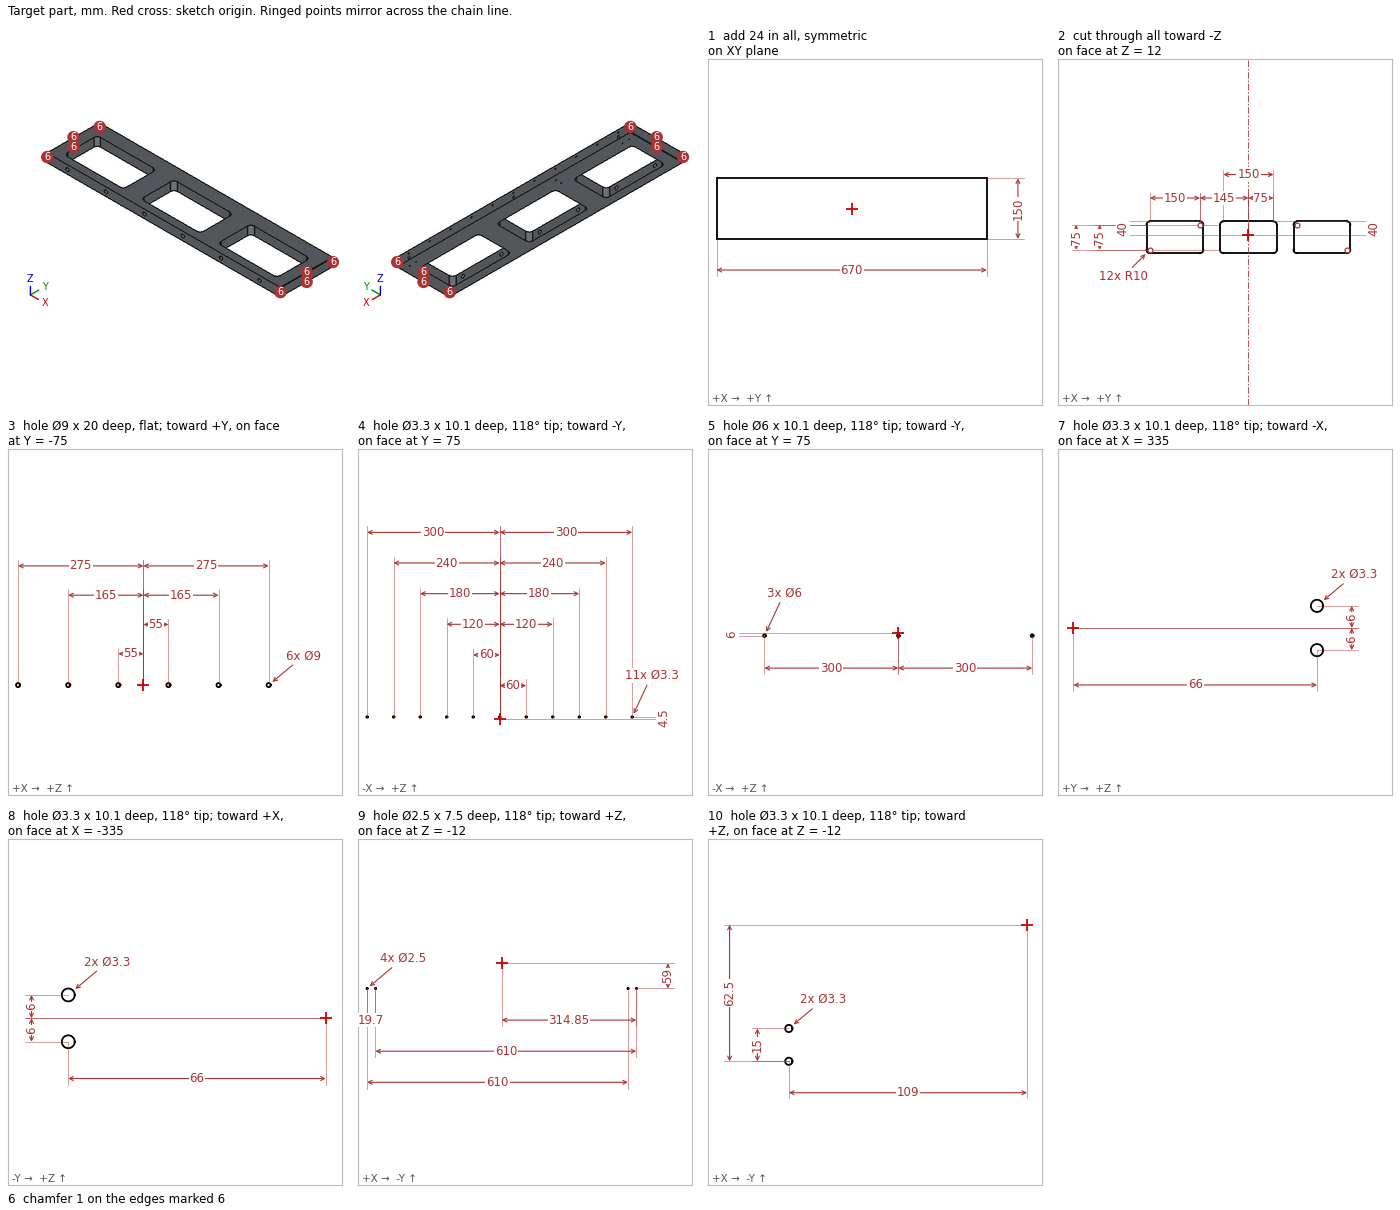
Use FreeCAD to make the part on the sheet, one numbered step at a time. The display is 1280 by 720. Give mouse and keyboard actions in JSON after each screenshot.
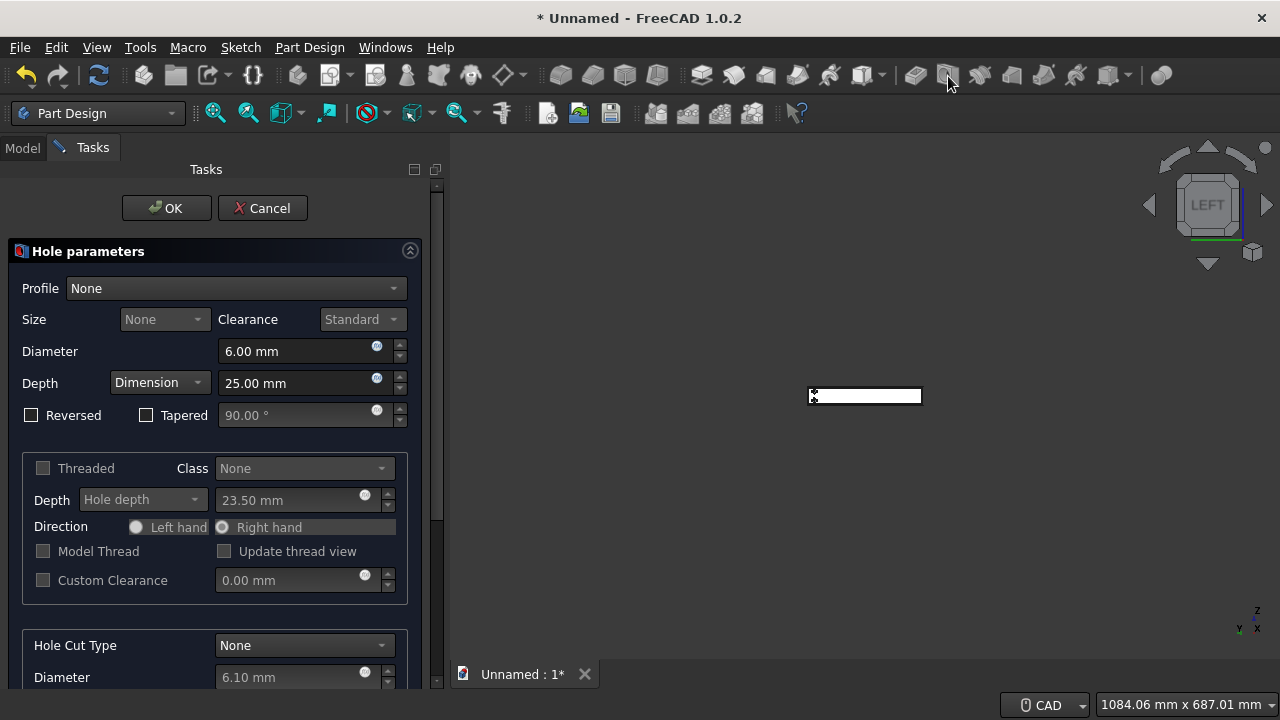
{"action": "triple_click", "coordinate": [305, 351]}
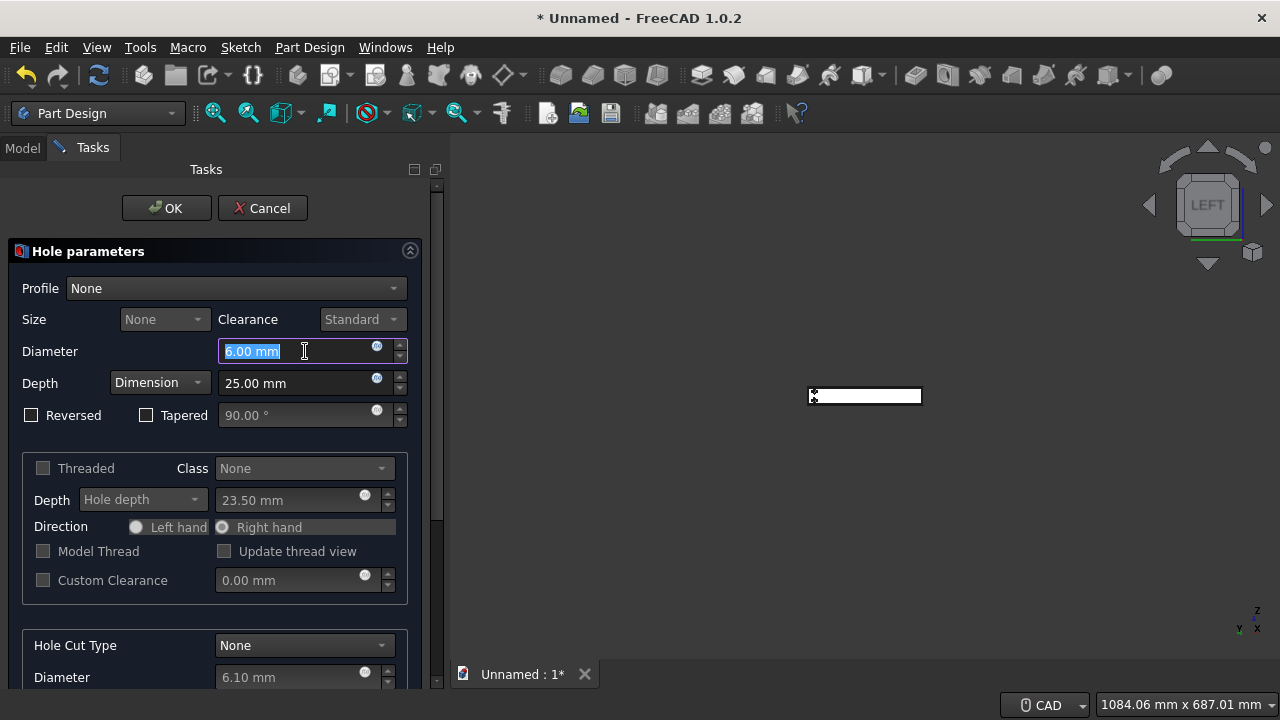
{"action": "type", "text": "3.3"}
{"action": "key", "text": "Tab"}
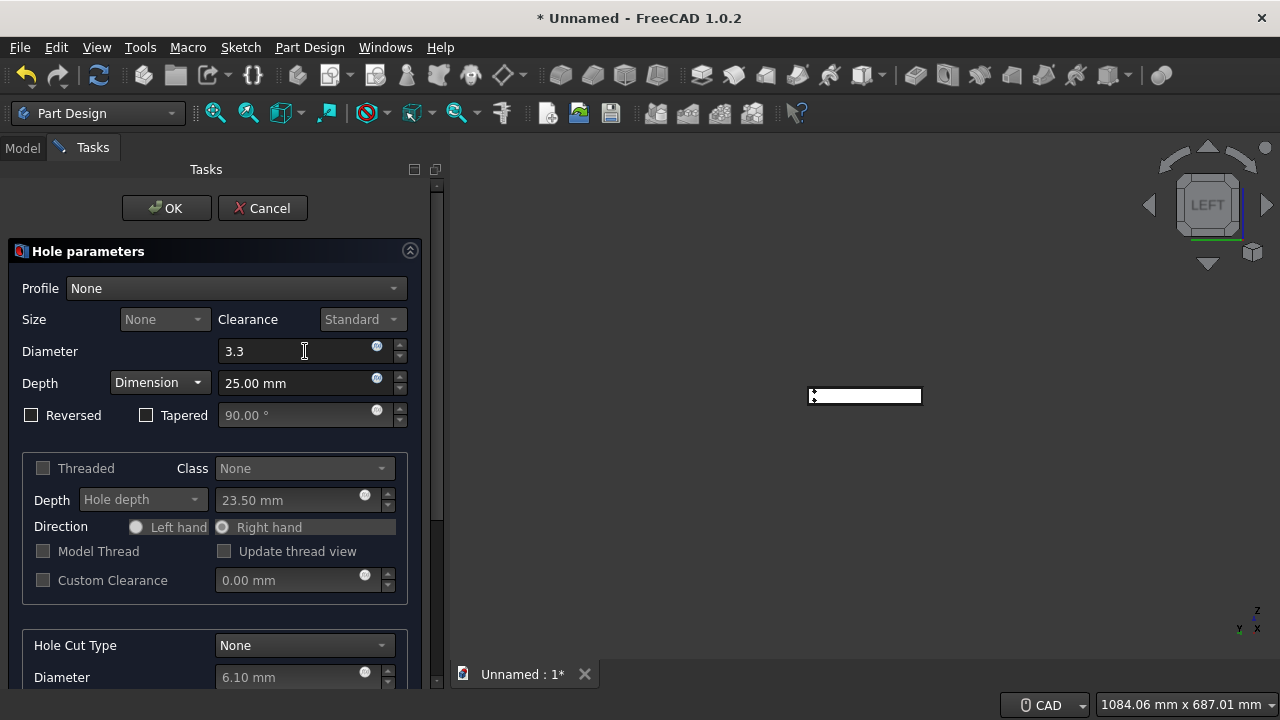
{"action": "triple_click", "coordinate": [305, 383]}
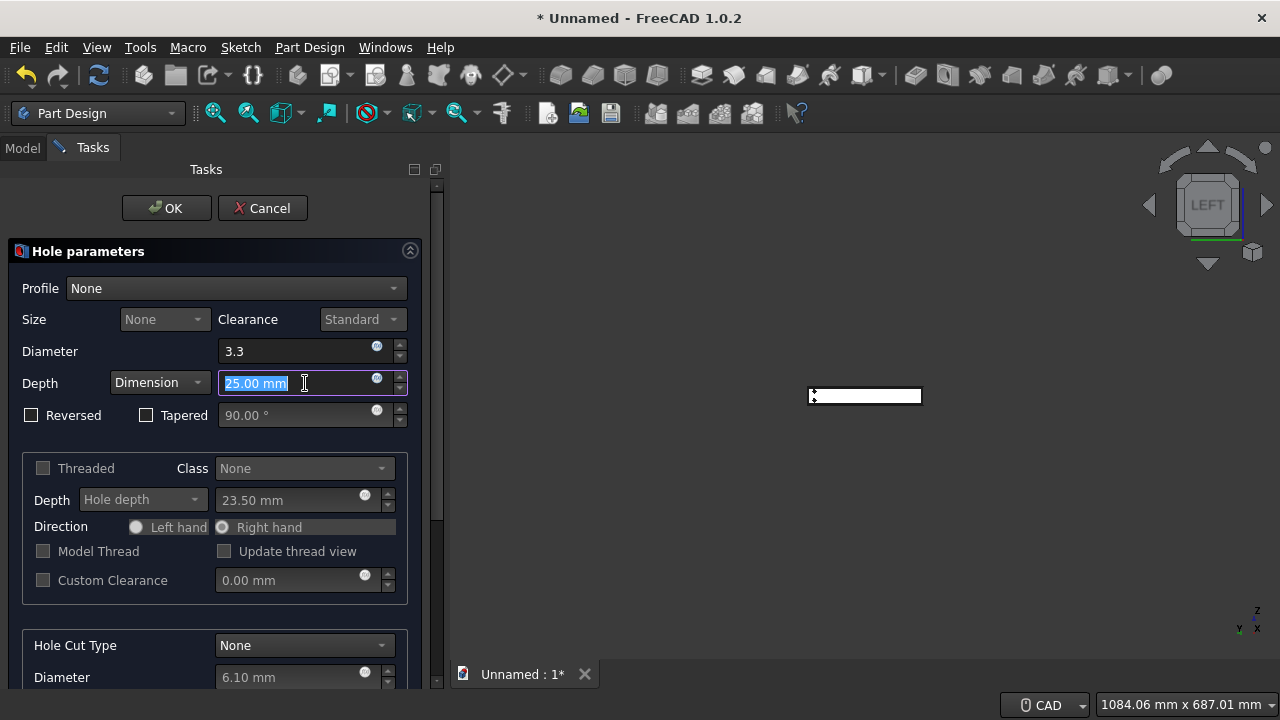
{"action": "type", "text": "10.1"}
{"action": "key", "text": "Tab"}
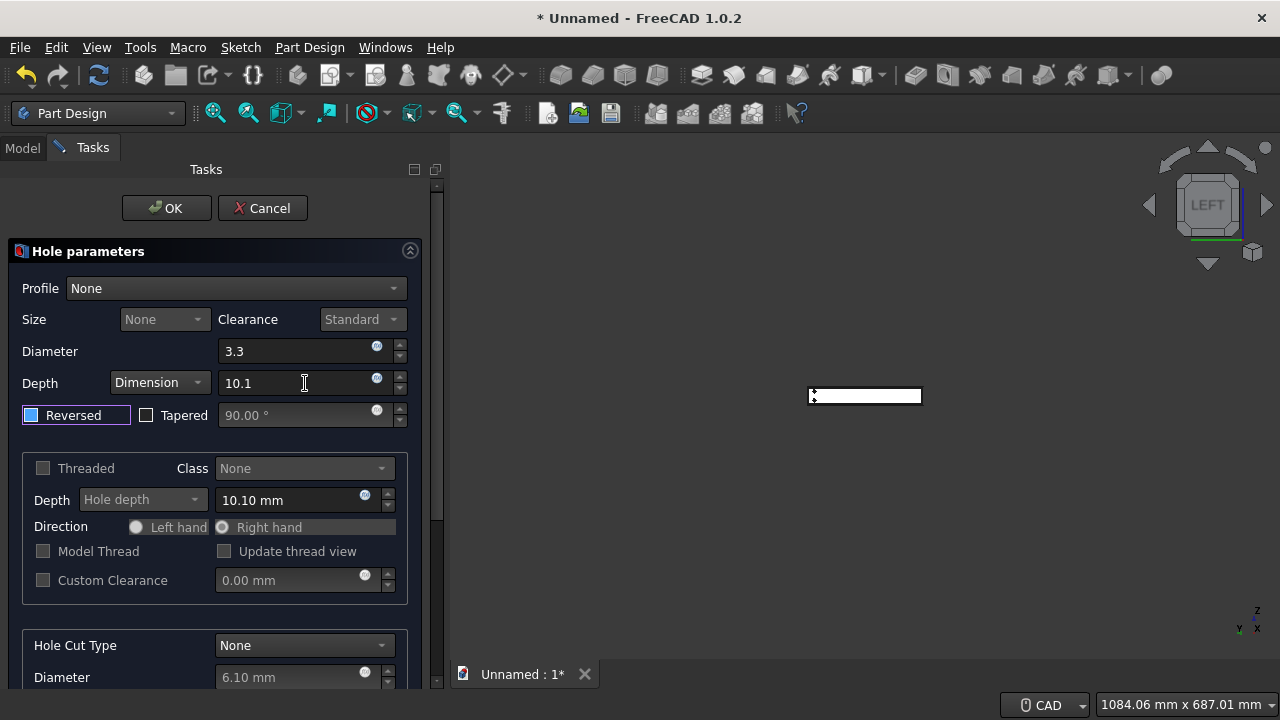
{"action": "left_click", "coordinate": [167, 208]}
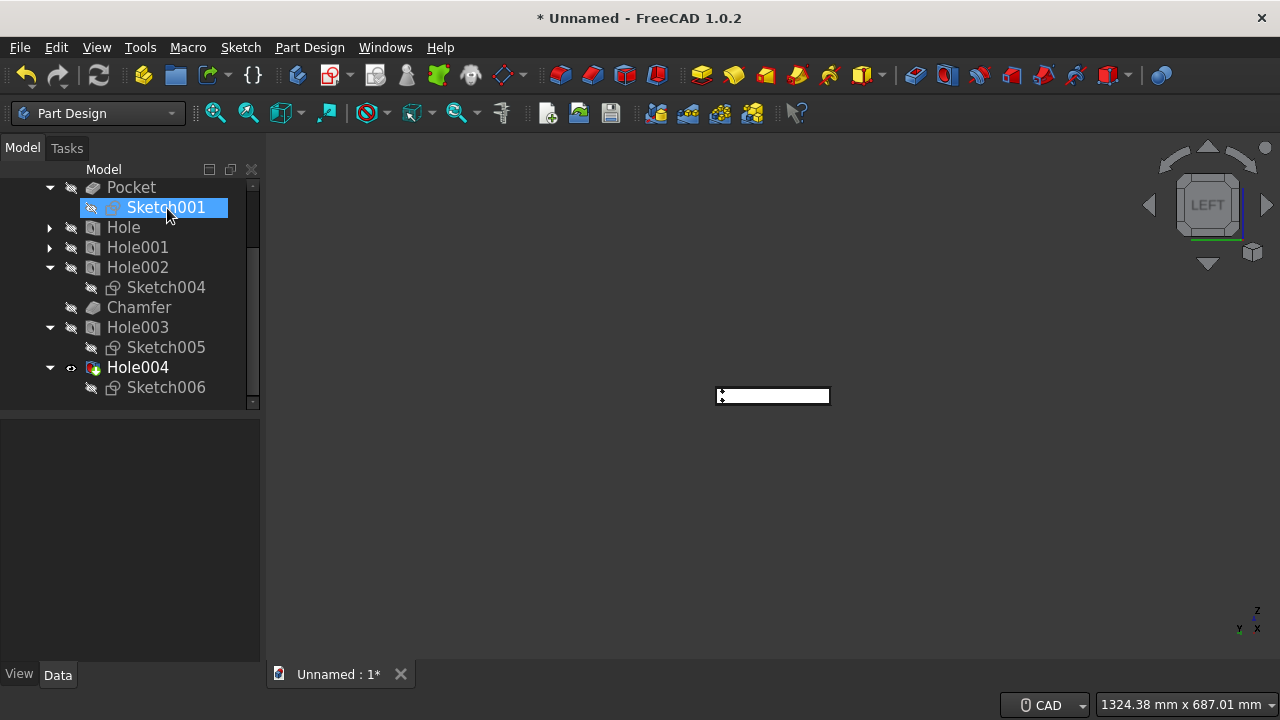
{"action": "key", "text": "v f"}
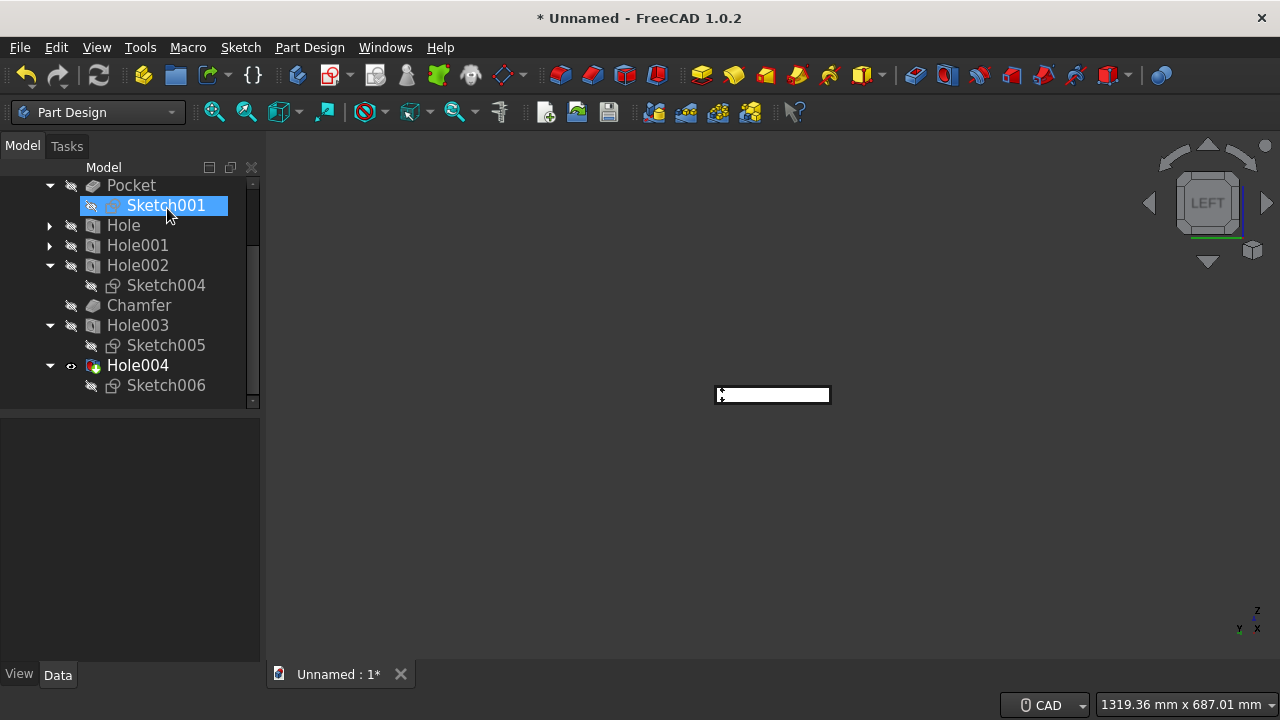
{"action": "key", "text": "5"}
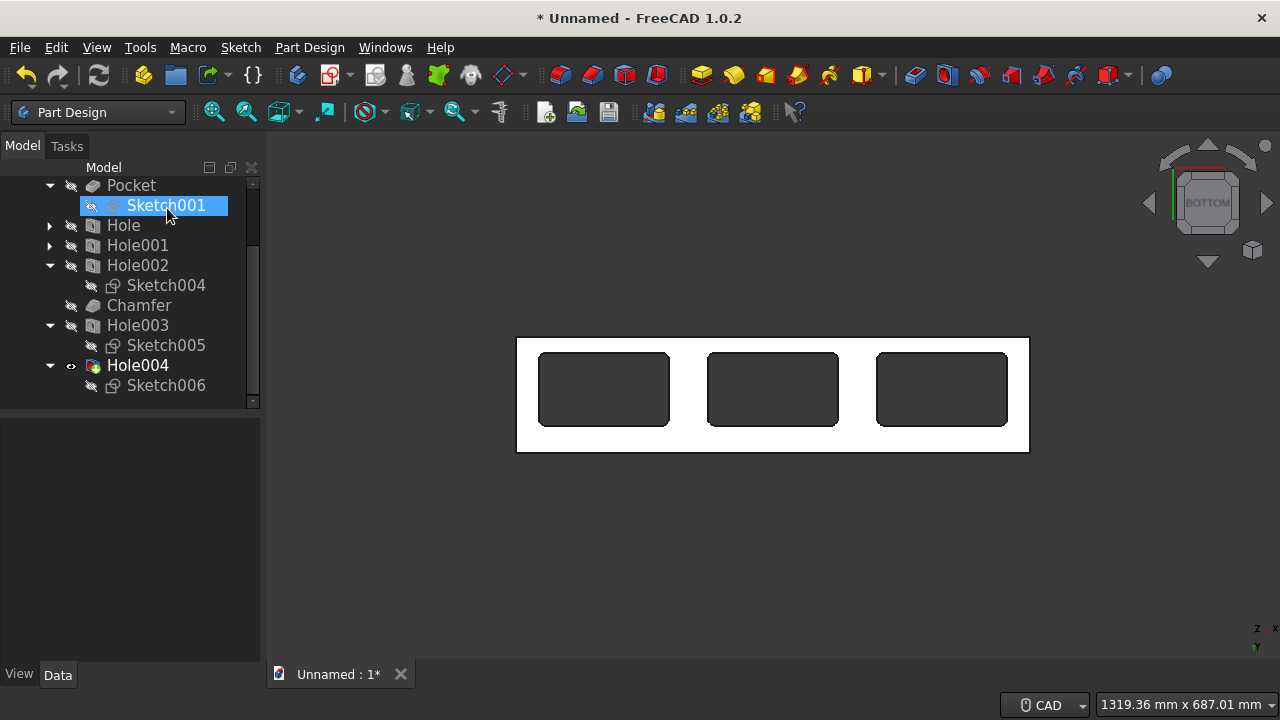
{"action": "left_click", "coordinate": [846, 427]}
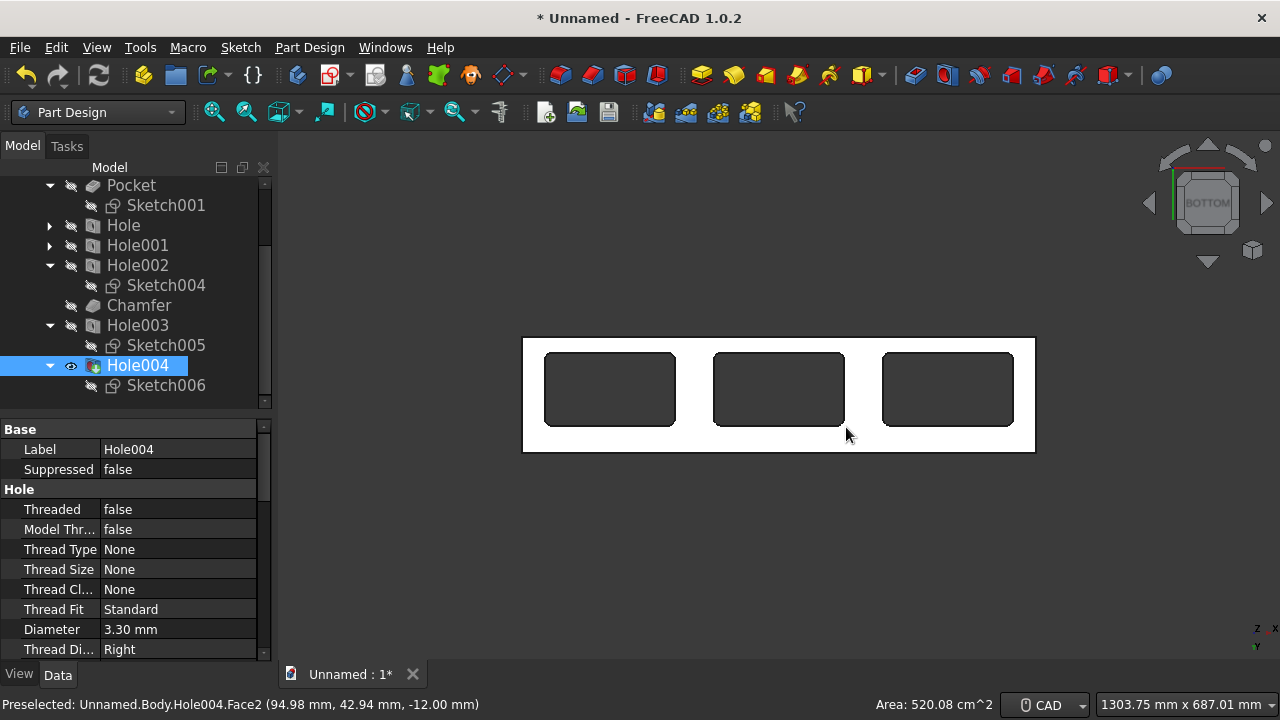
{"action": "left_click", "coordinate": [330, 76]}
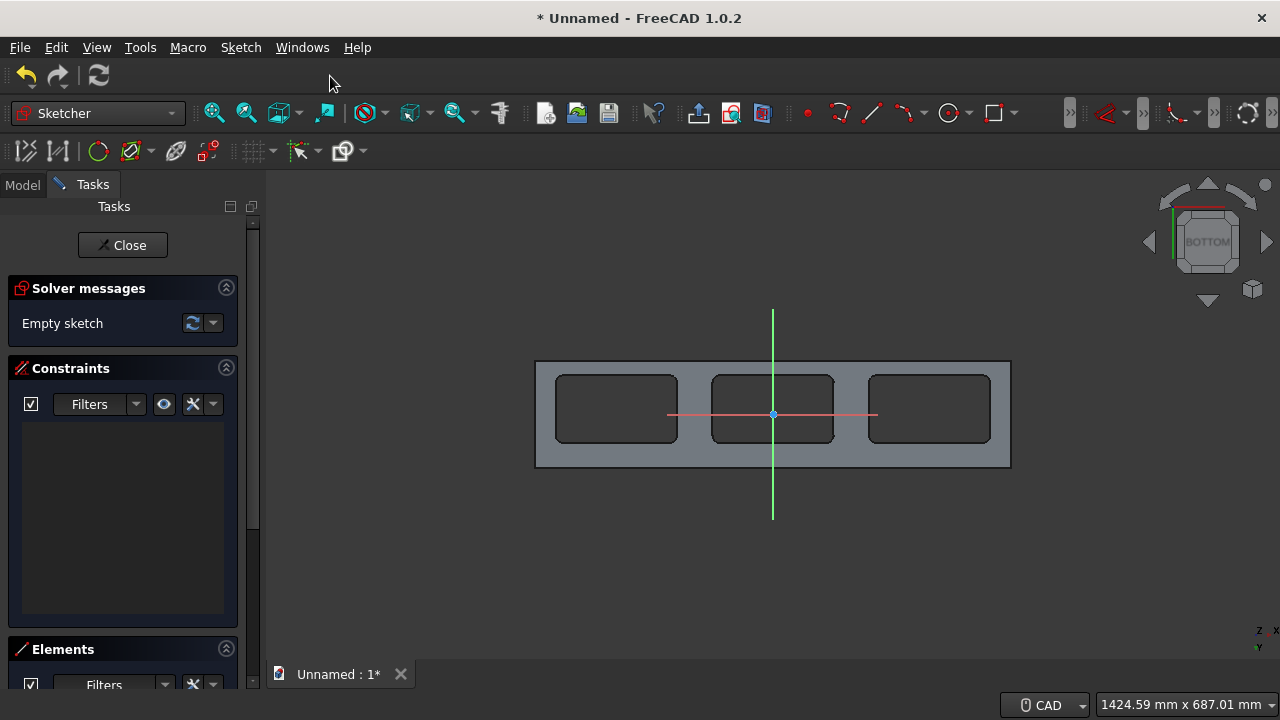
{"action": "left_click", "coordinate": [950, 114]}